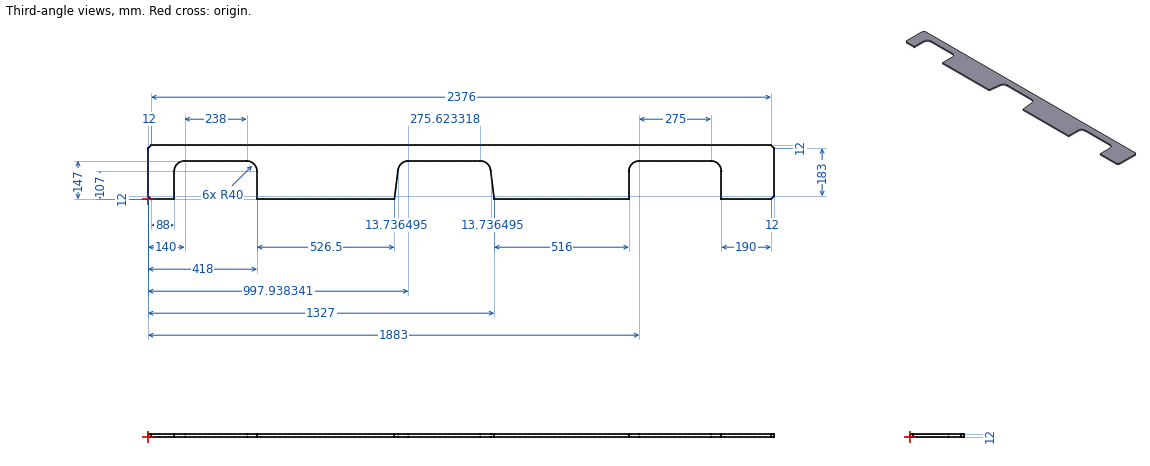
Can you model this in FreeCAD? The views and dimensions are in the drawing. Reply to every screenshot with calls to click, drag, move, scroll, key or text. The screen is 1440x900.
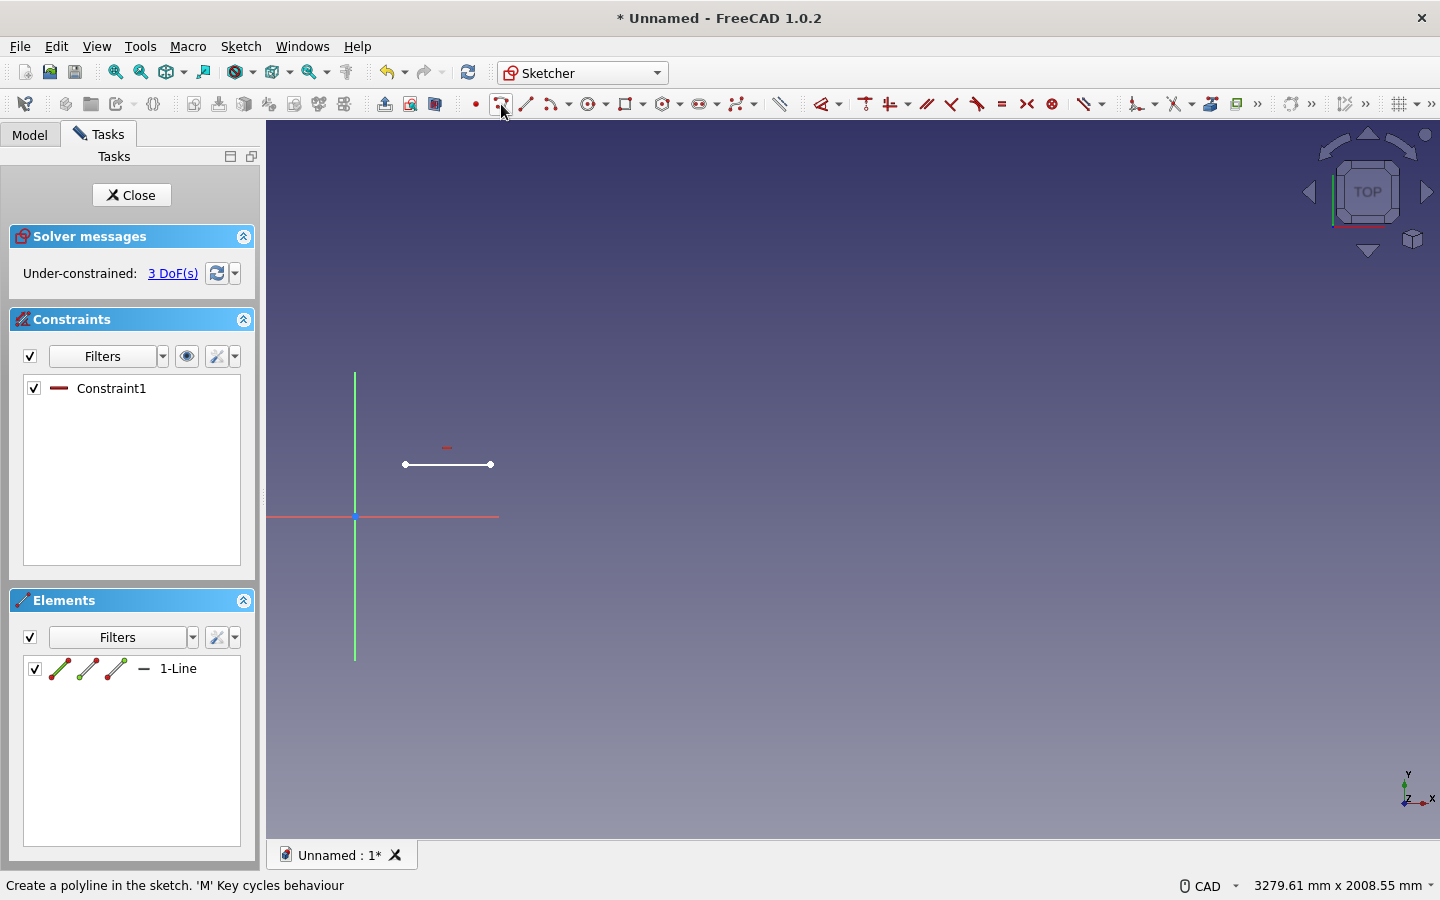
click(505, 478)
click(505, 517)
click(693, 508)
click(698, 477)
right_click(698, 477)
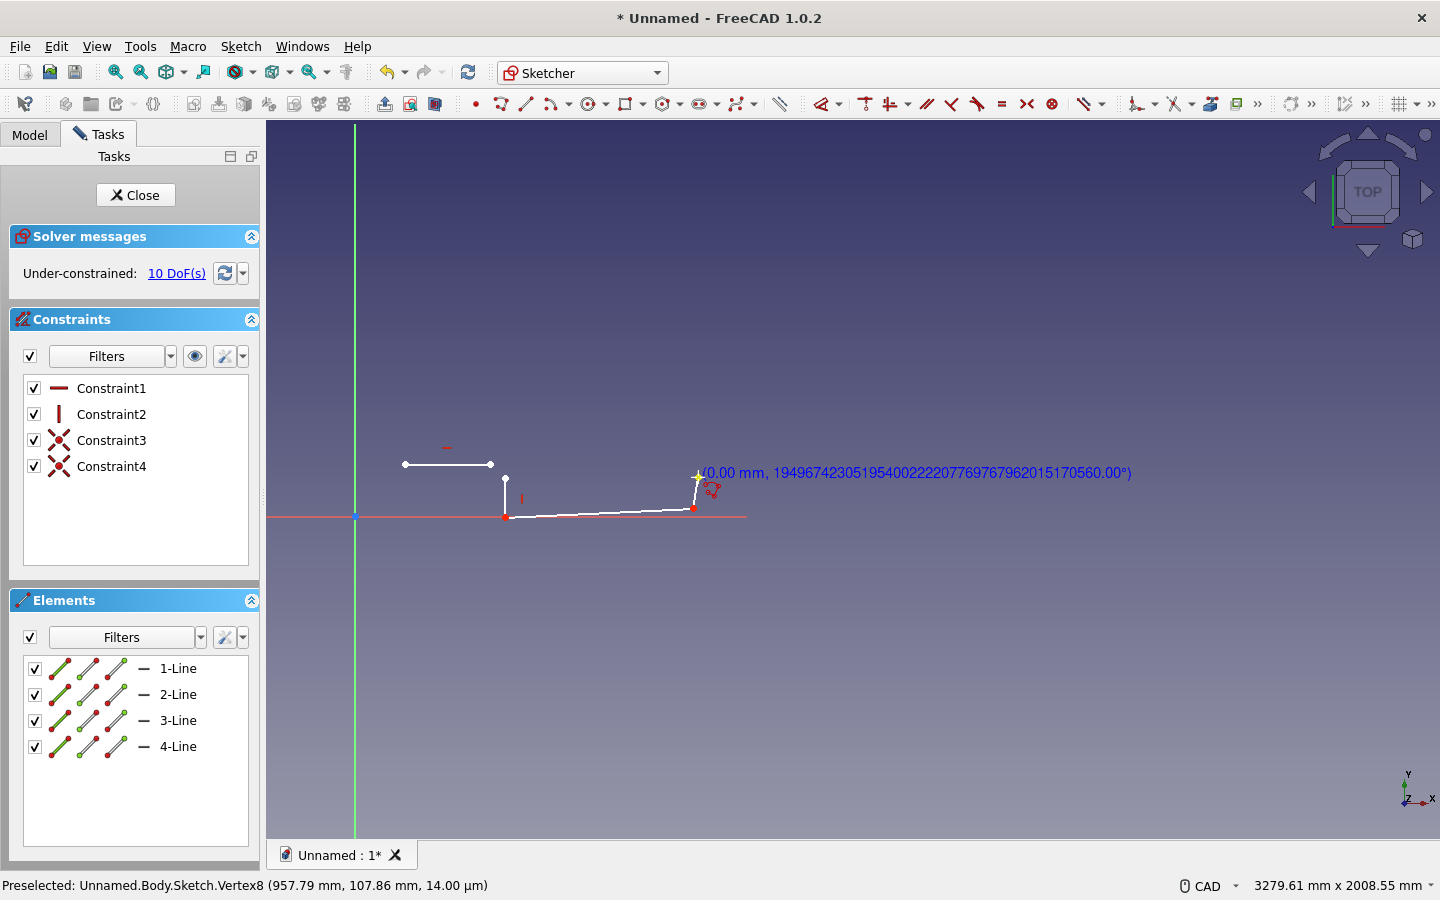
click(526, 104)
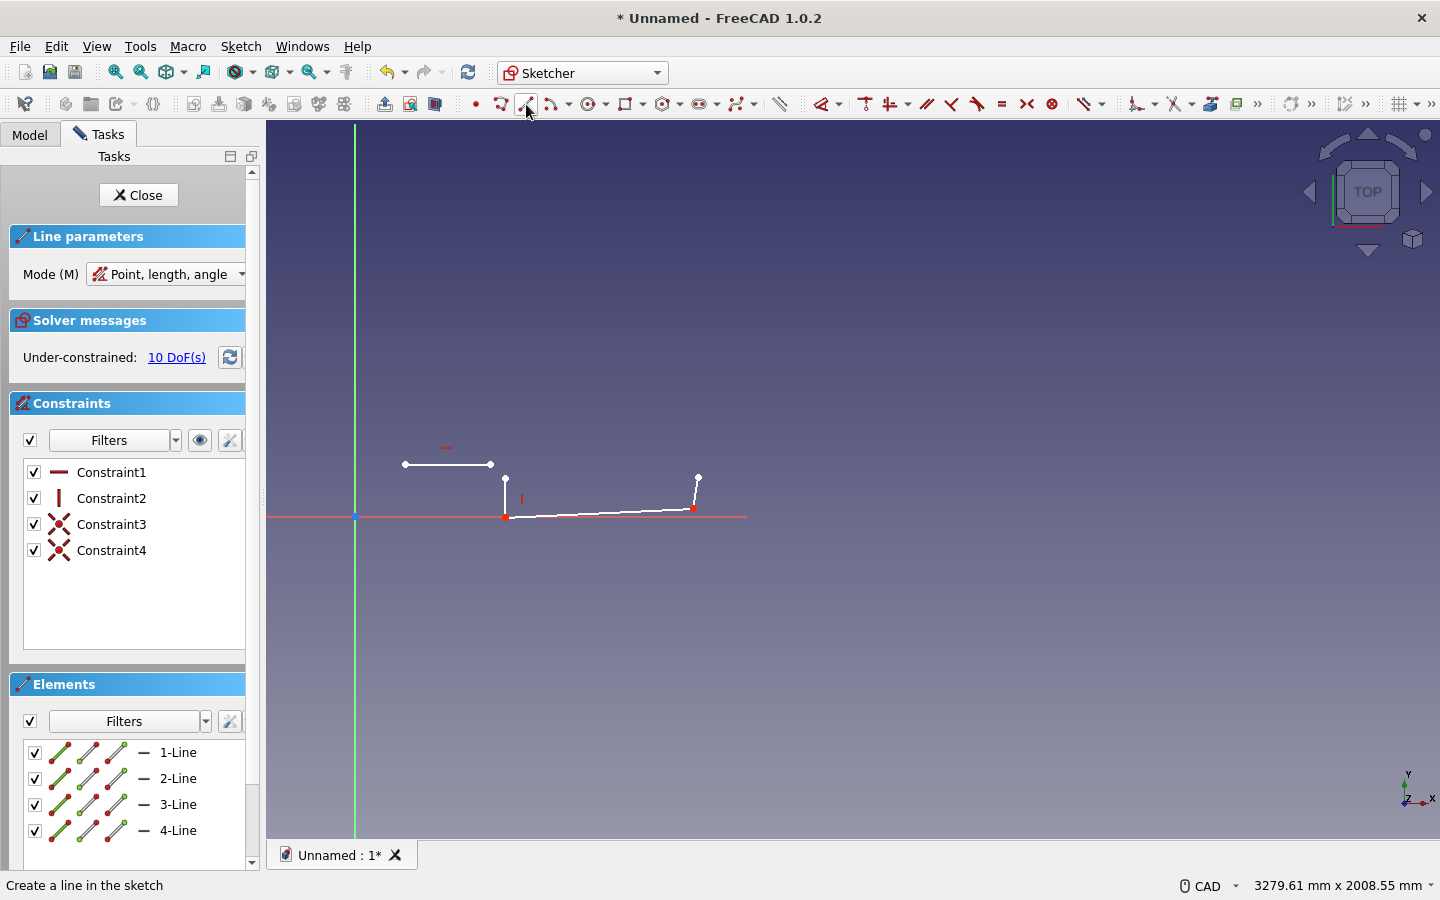
click(712, 464)
click(811, 464)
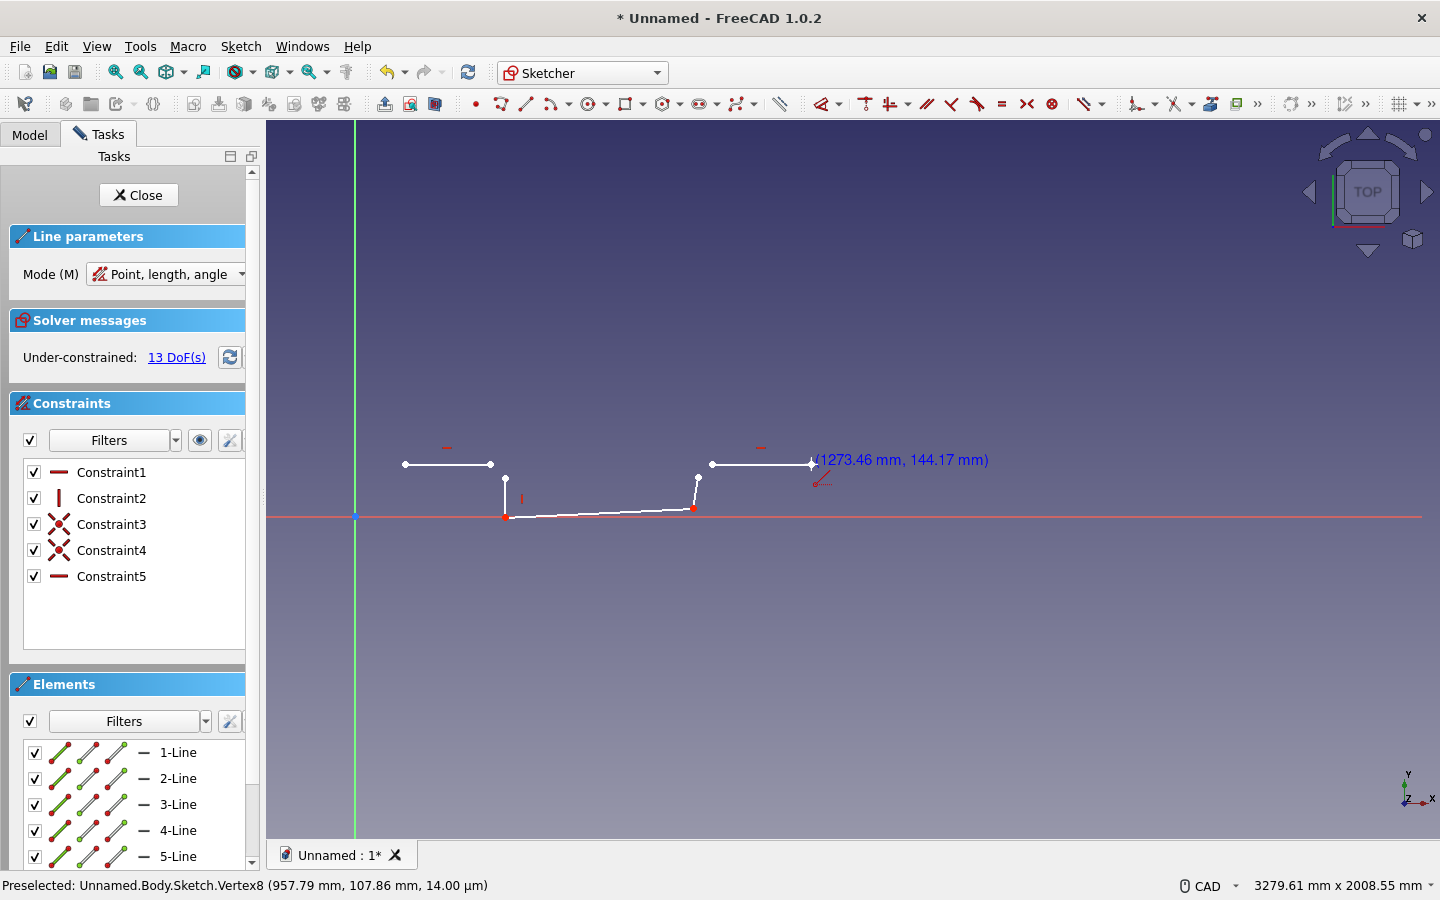
click(501, 104)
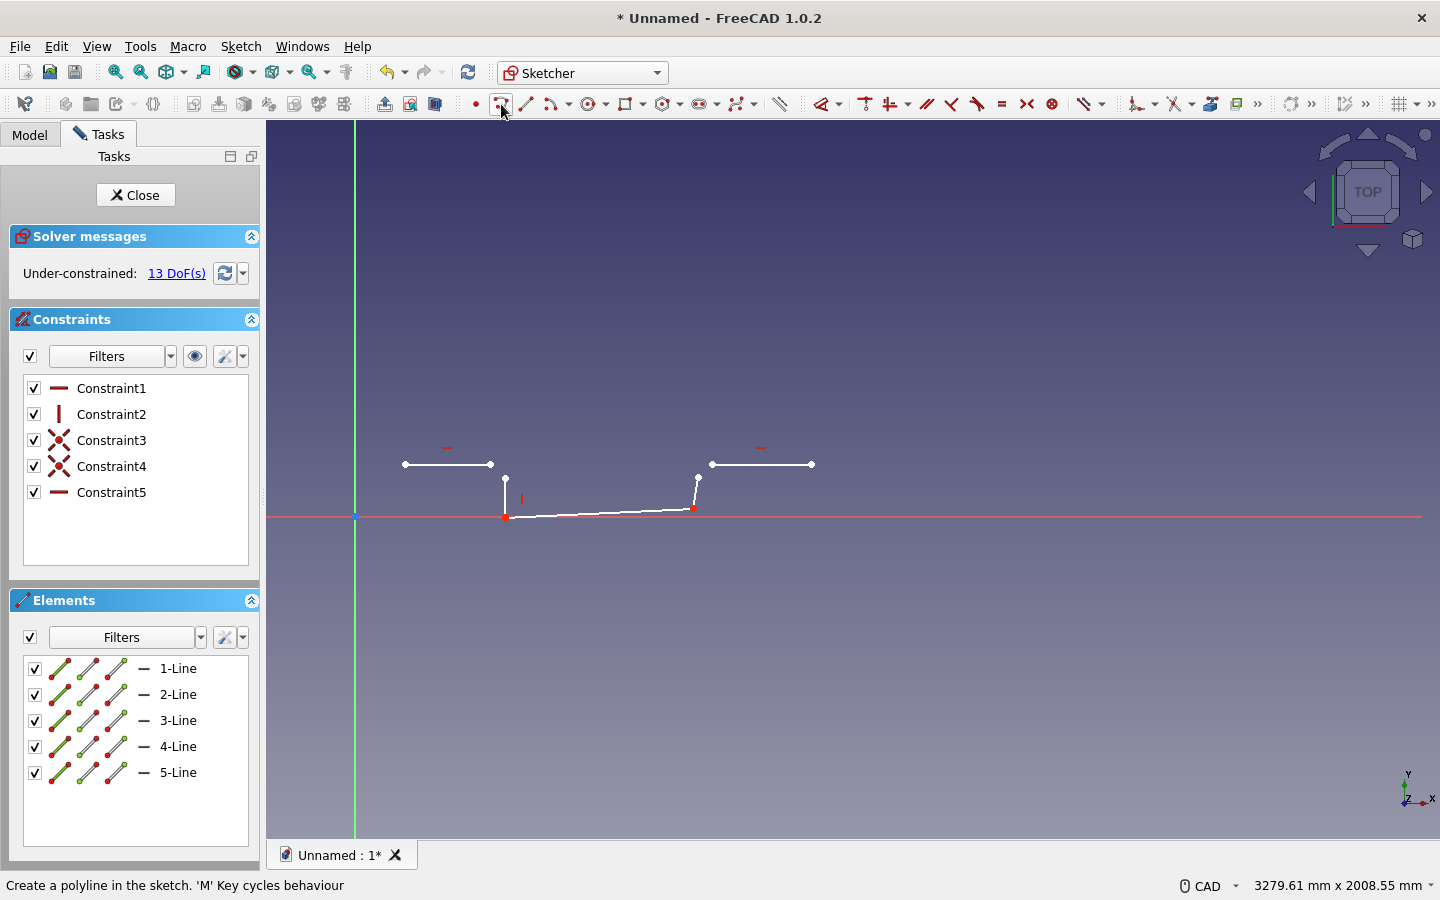
click(825, 477)
click(830, 517)
click(1015, 508)
click(1015, 478)
right_click(1015, 478)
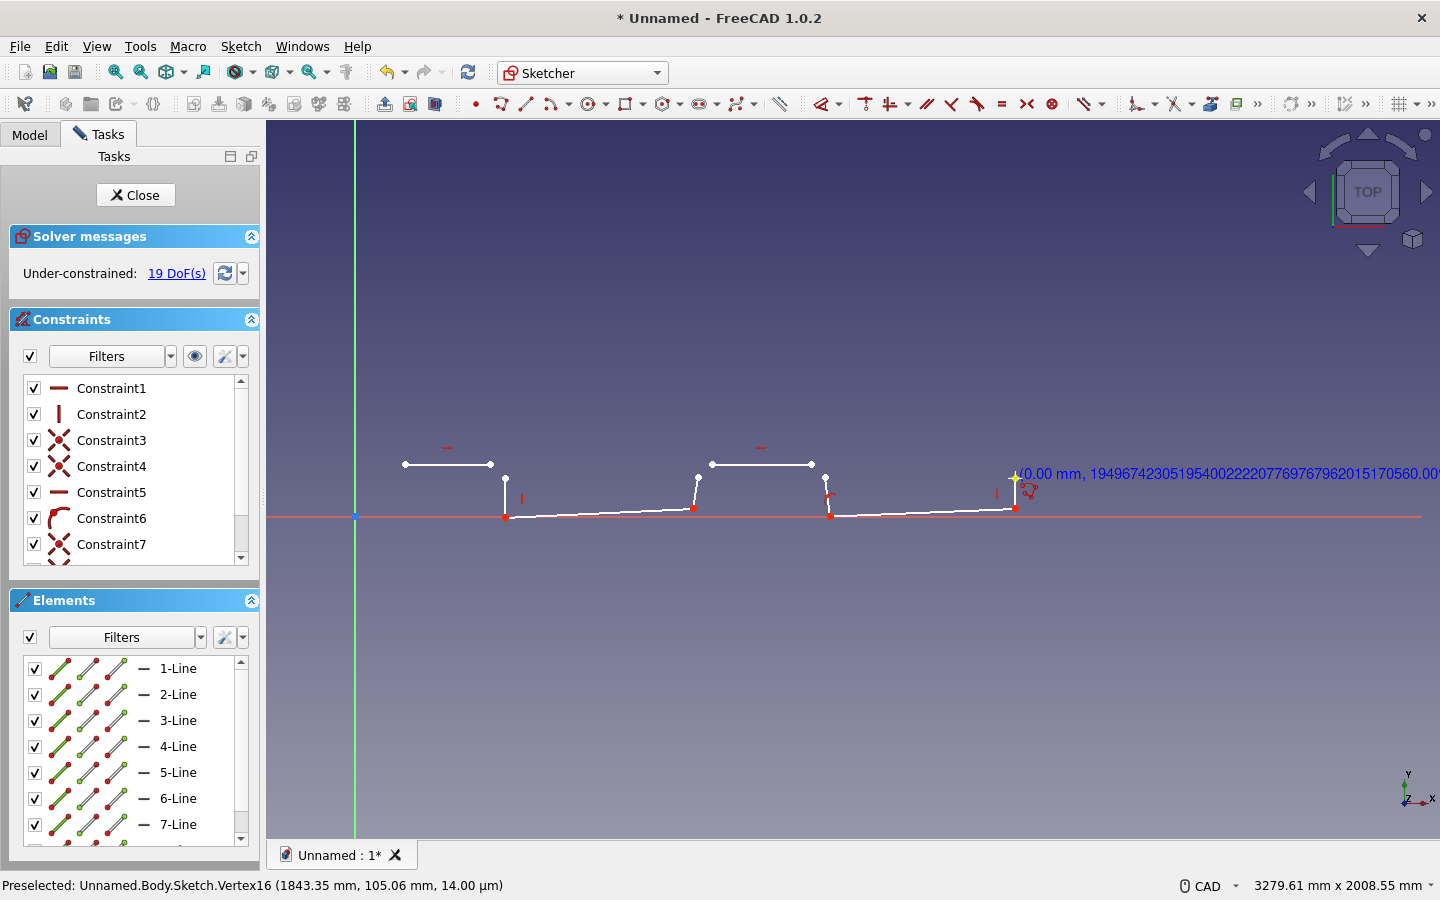
click(526, 104)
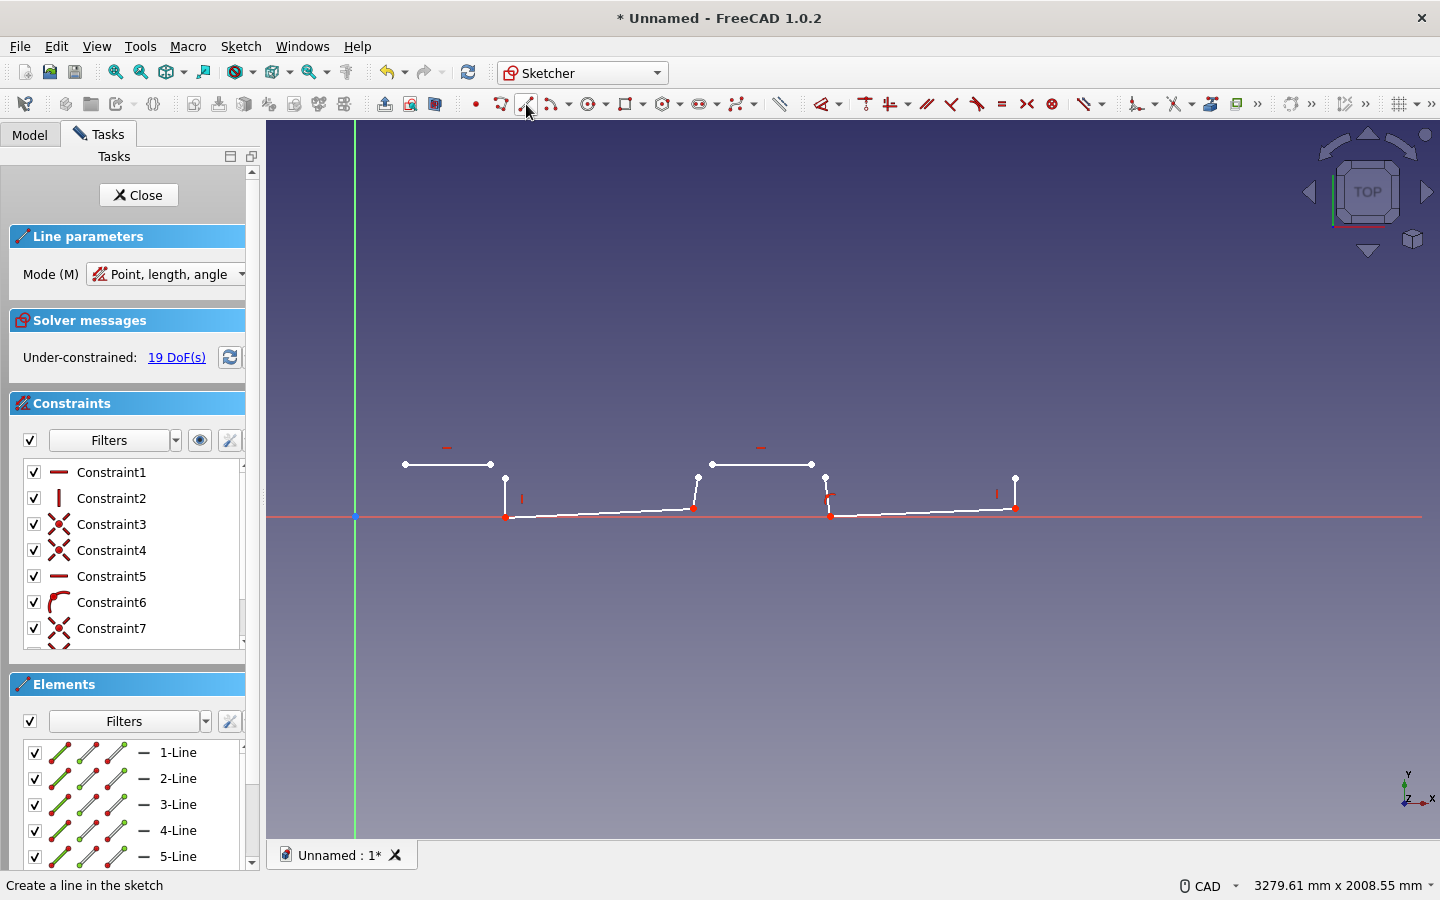
click(1029, 464)
click(1128, 464)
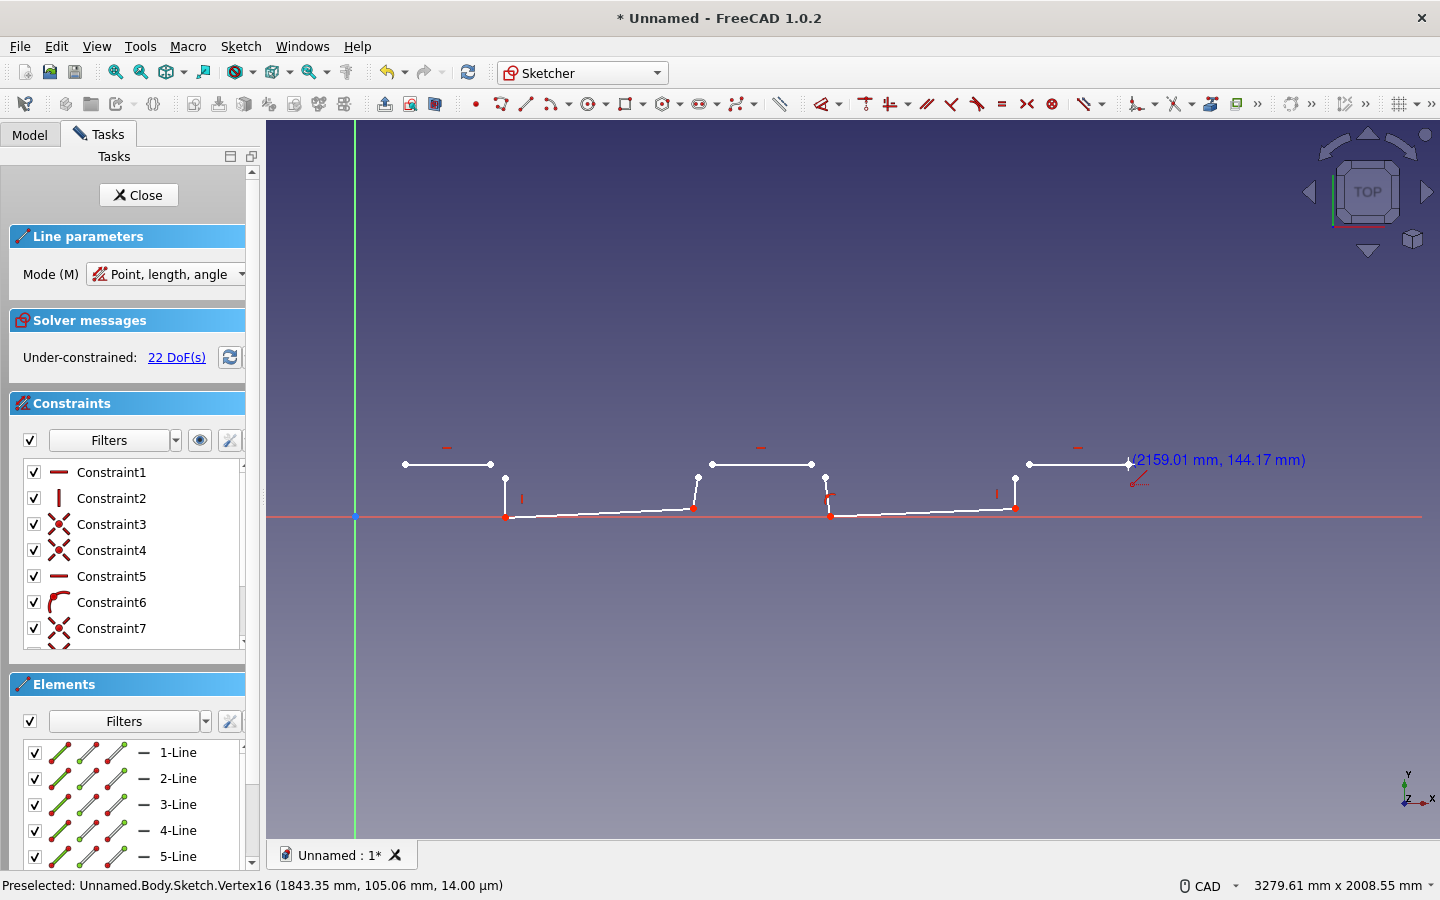
click(501, 104)